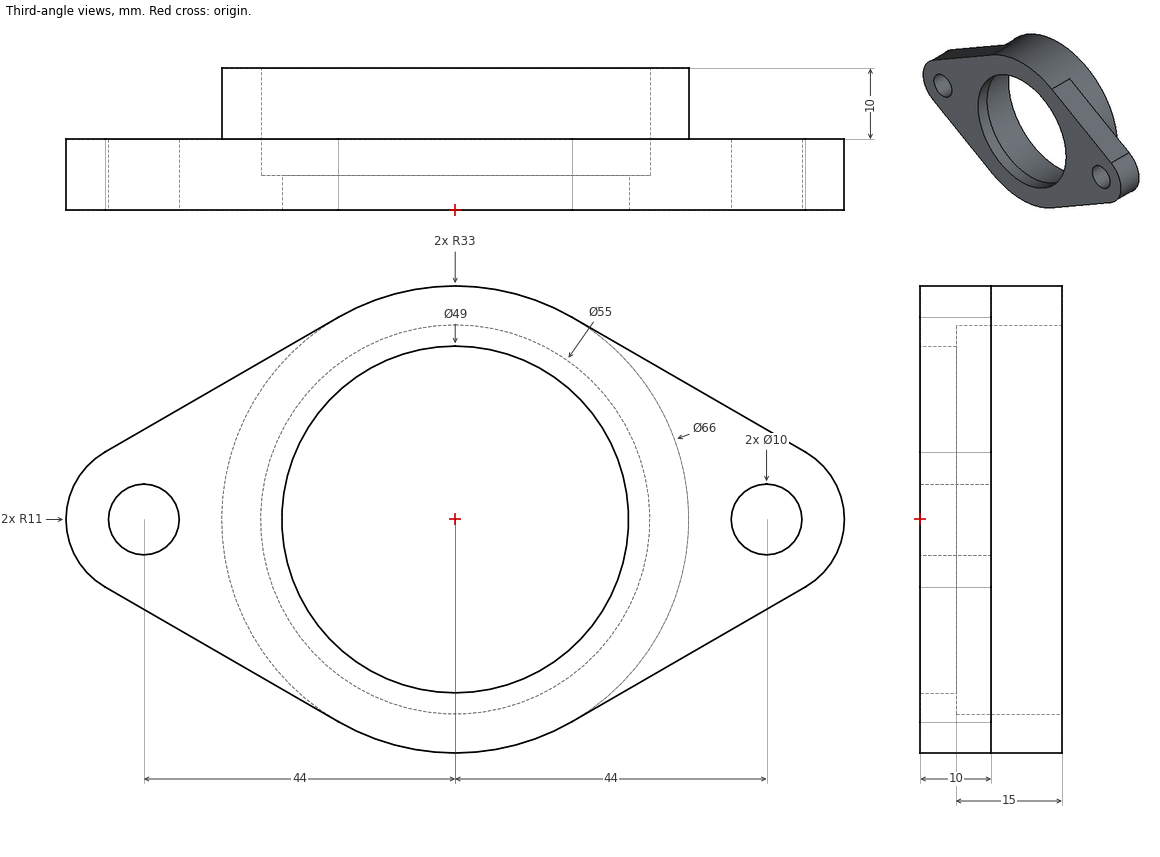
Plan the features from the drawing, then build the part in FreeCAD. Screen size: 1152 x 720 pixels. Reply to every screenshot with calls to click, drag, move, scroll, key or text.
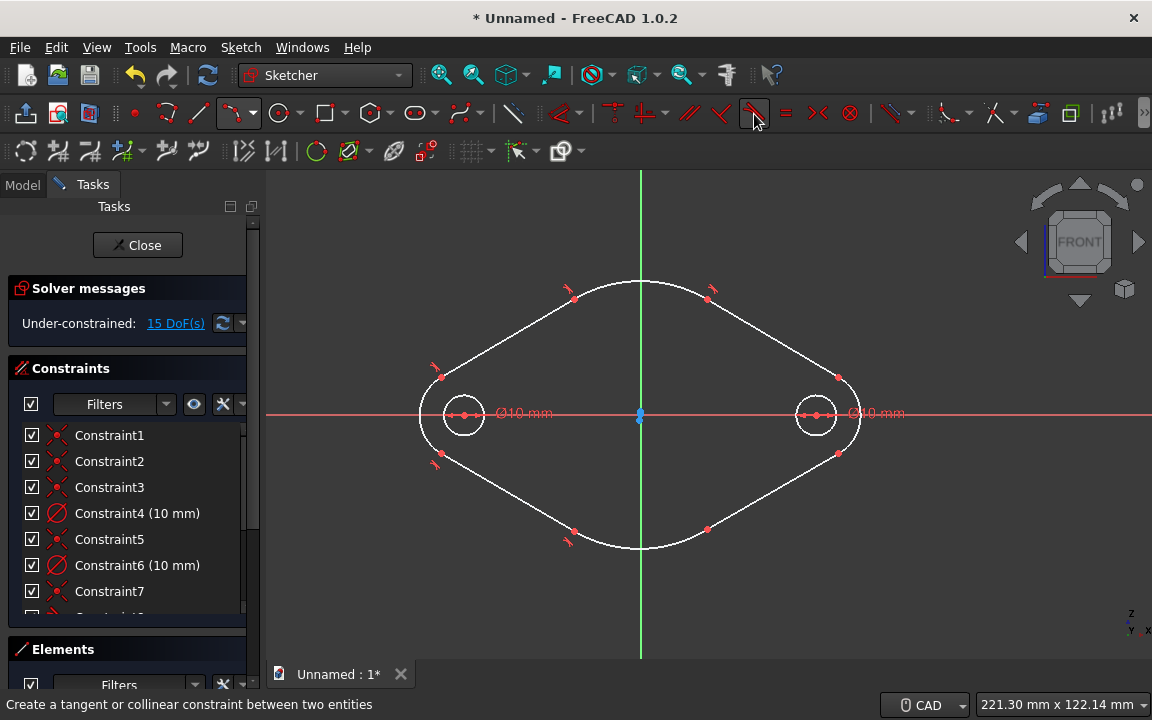
click(746, 323)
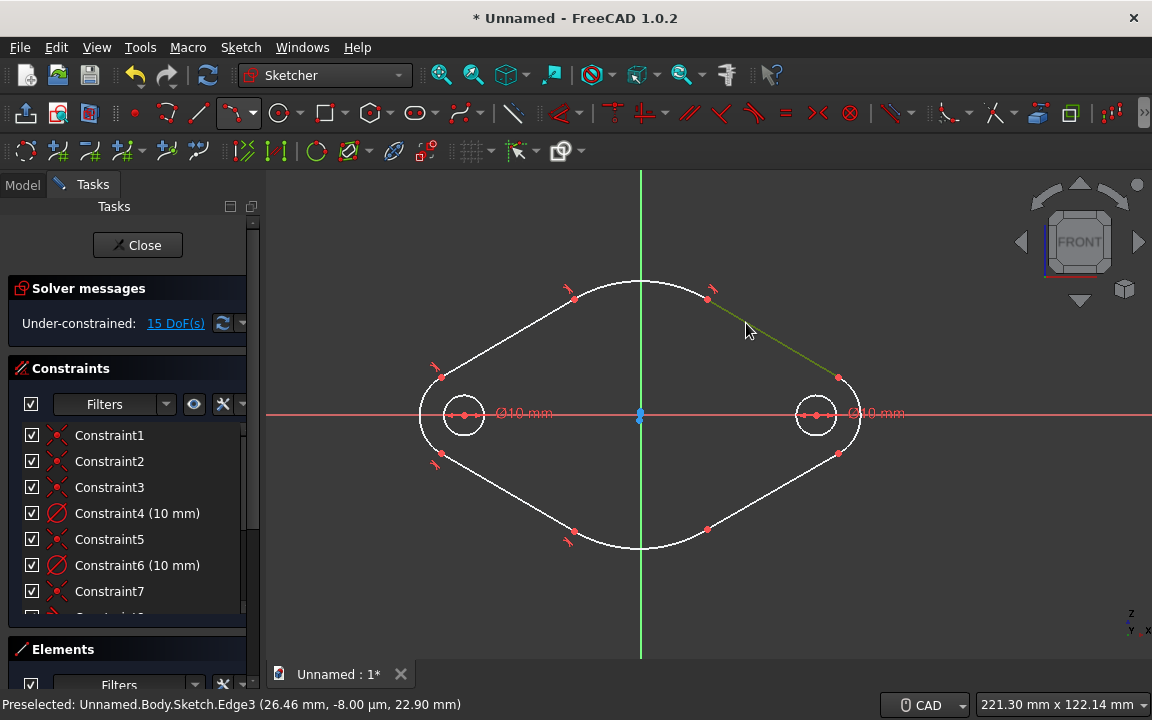
click(857, 434)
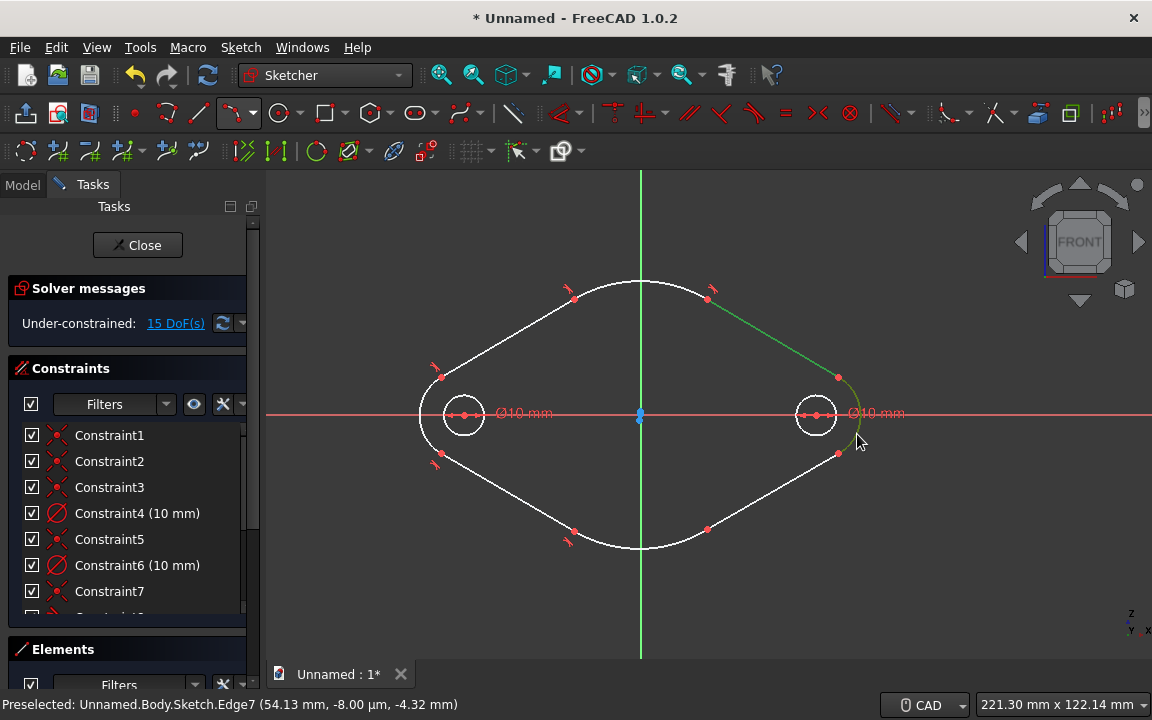
click(754, 114)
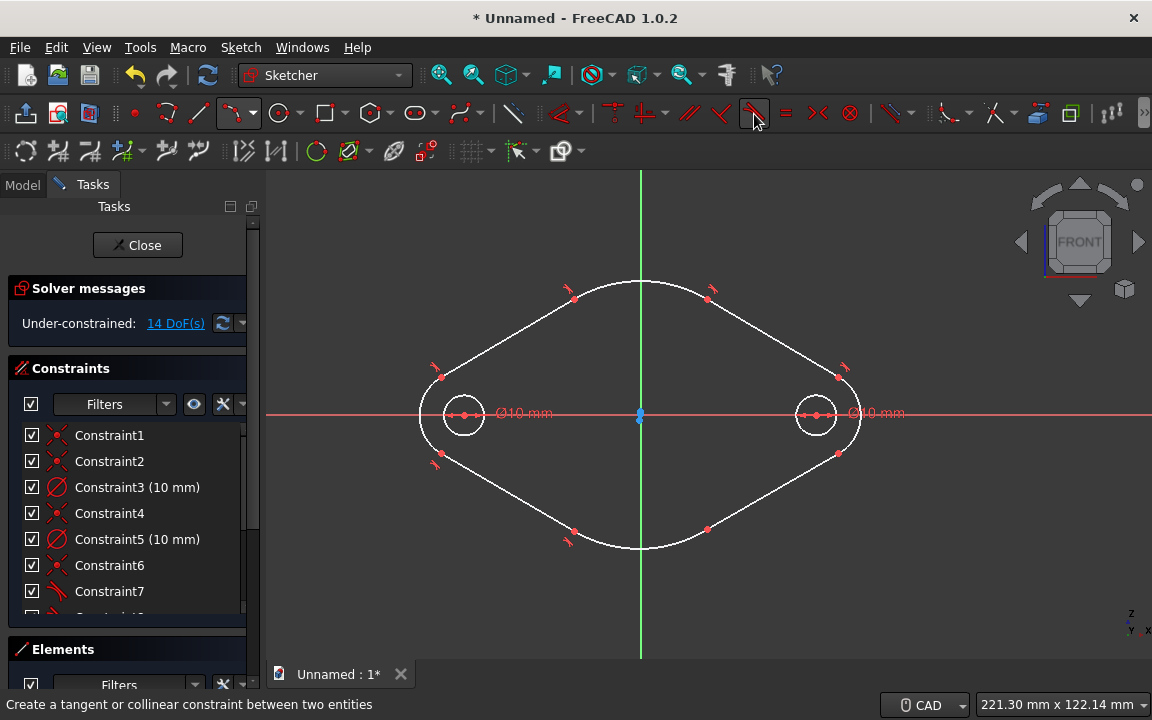
click(799, 477)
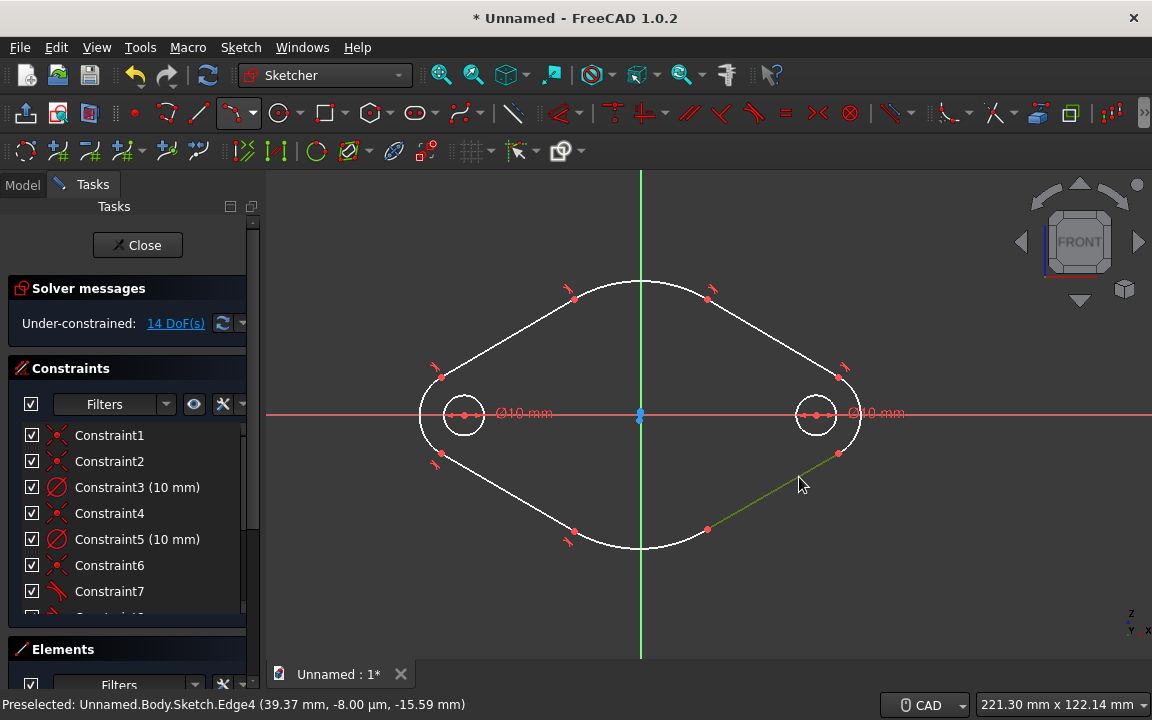
click(857, 434)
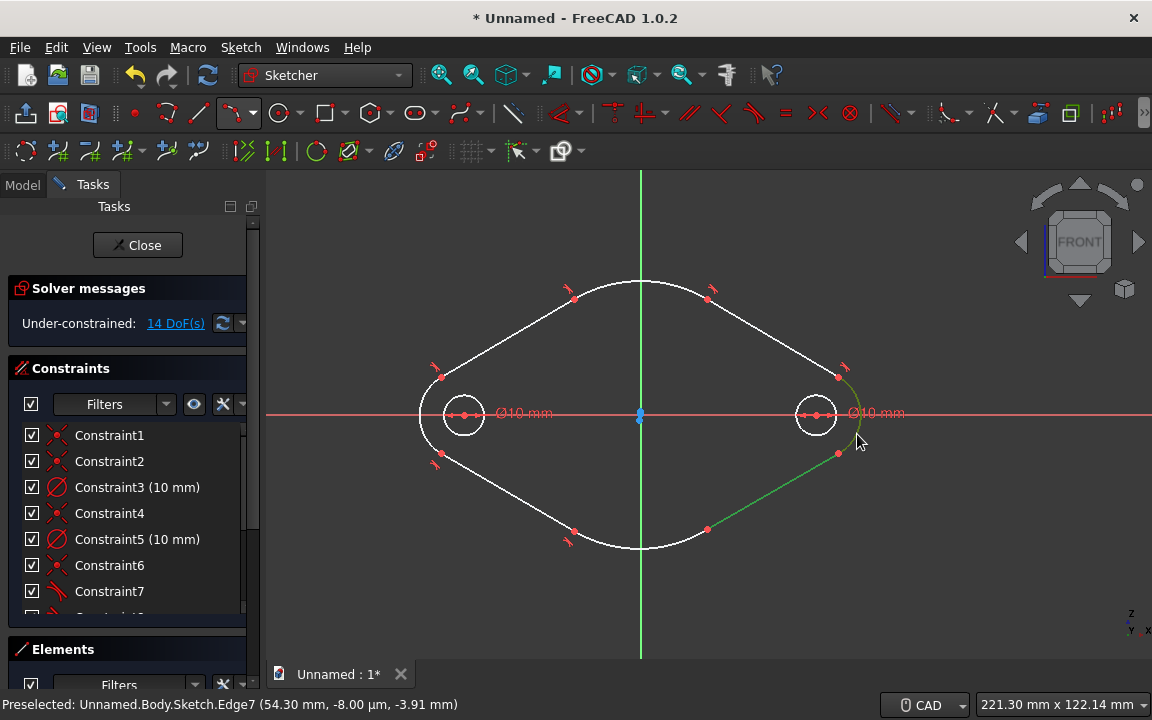
click(754, 114)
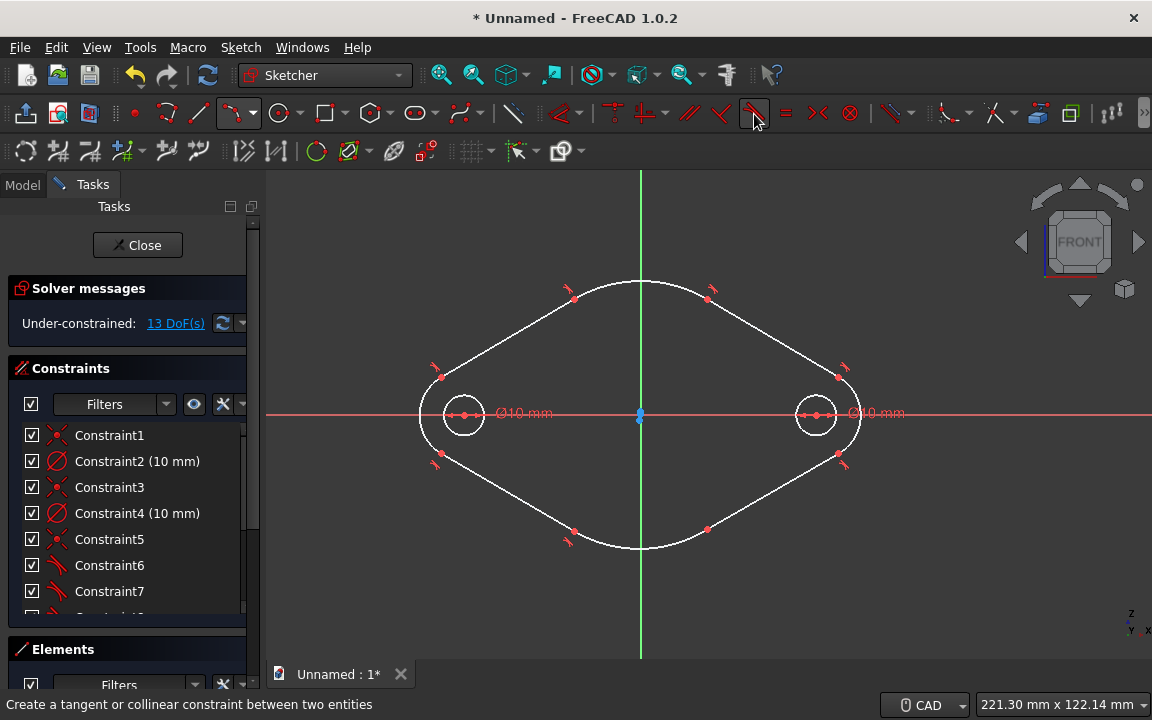
click(799, 477)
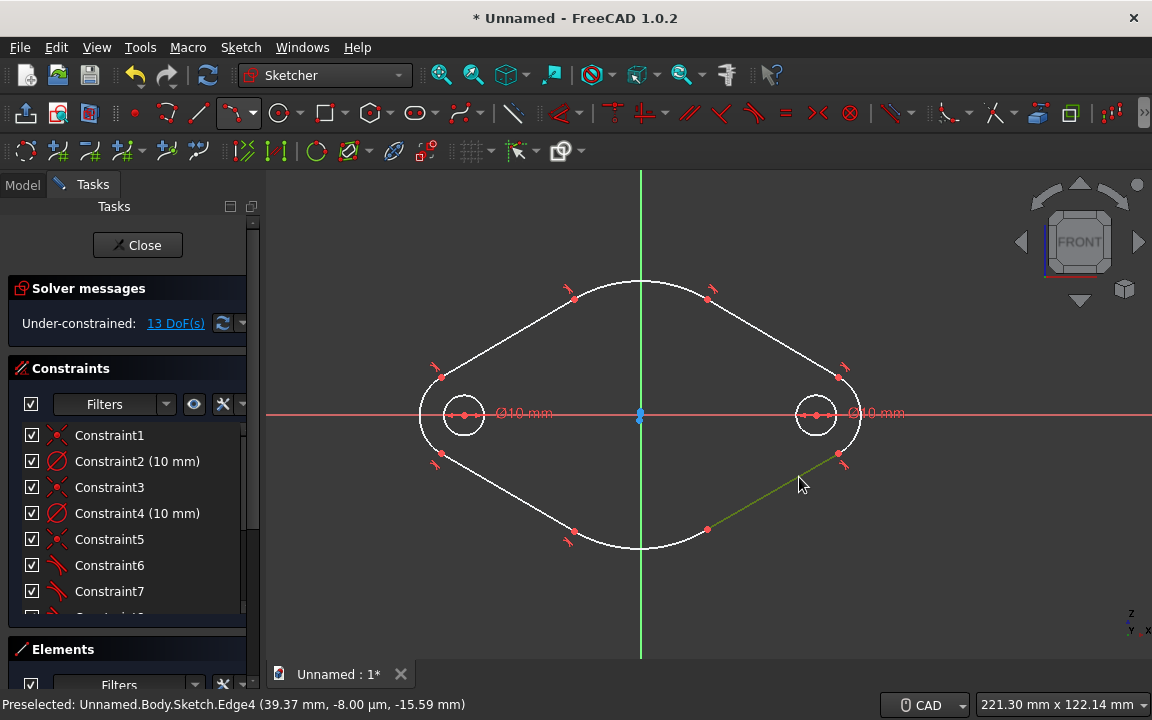
click(613, 546)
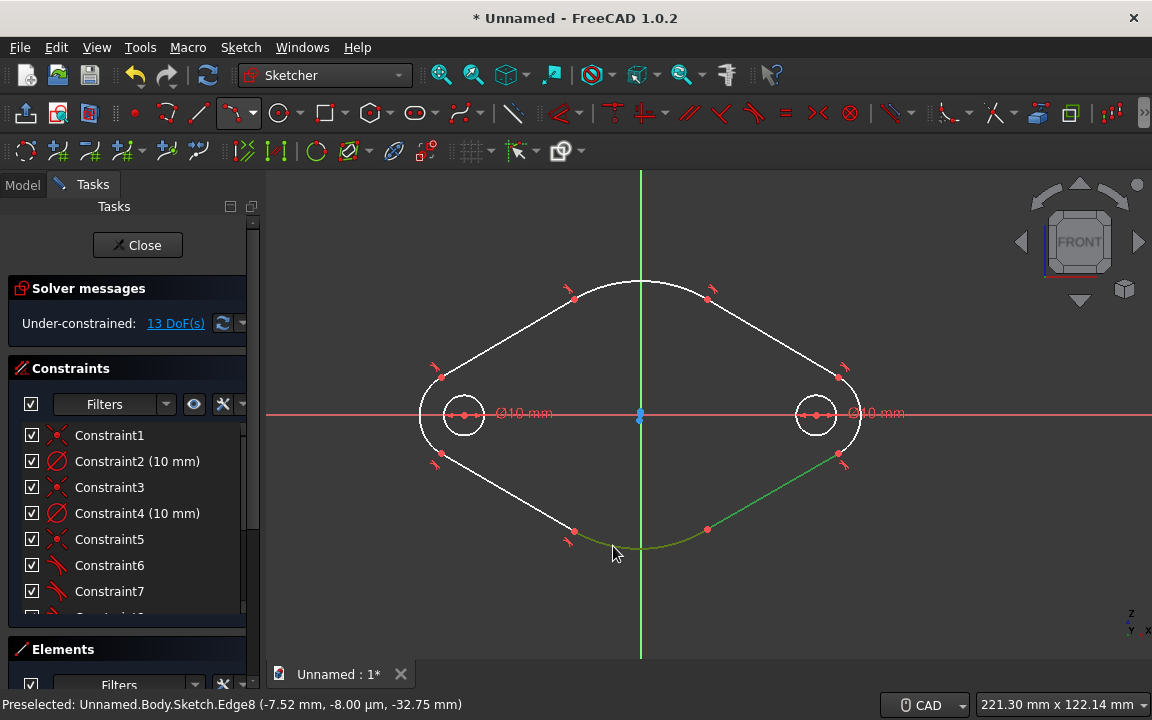
click(754, 114)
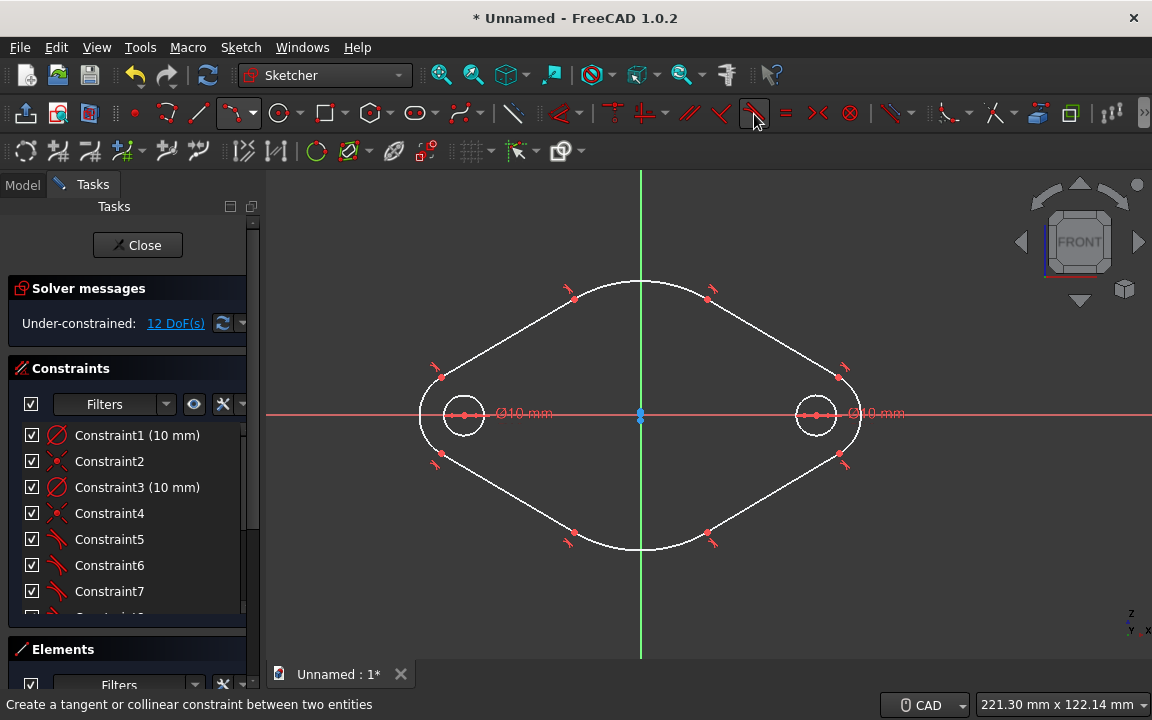
click(668, 284)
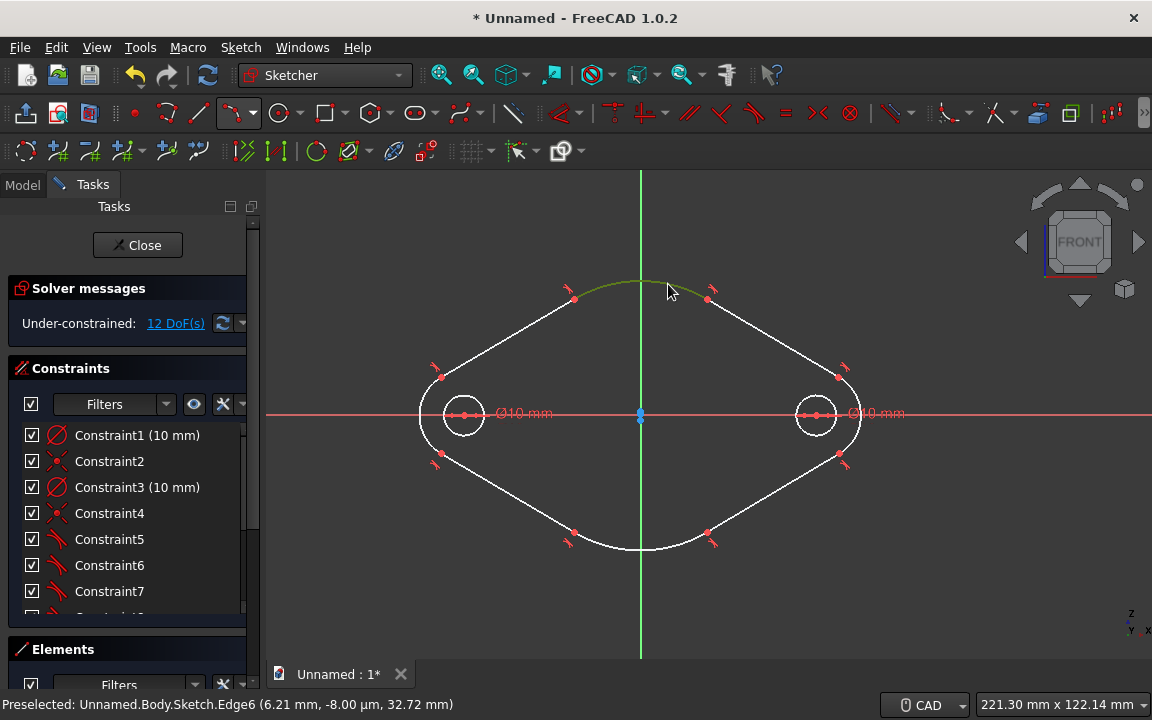
click(613, 548)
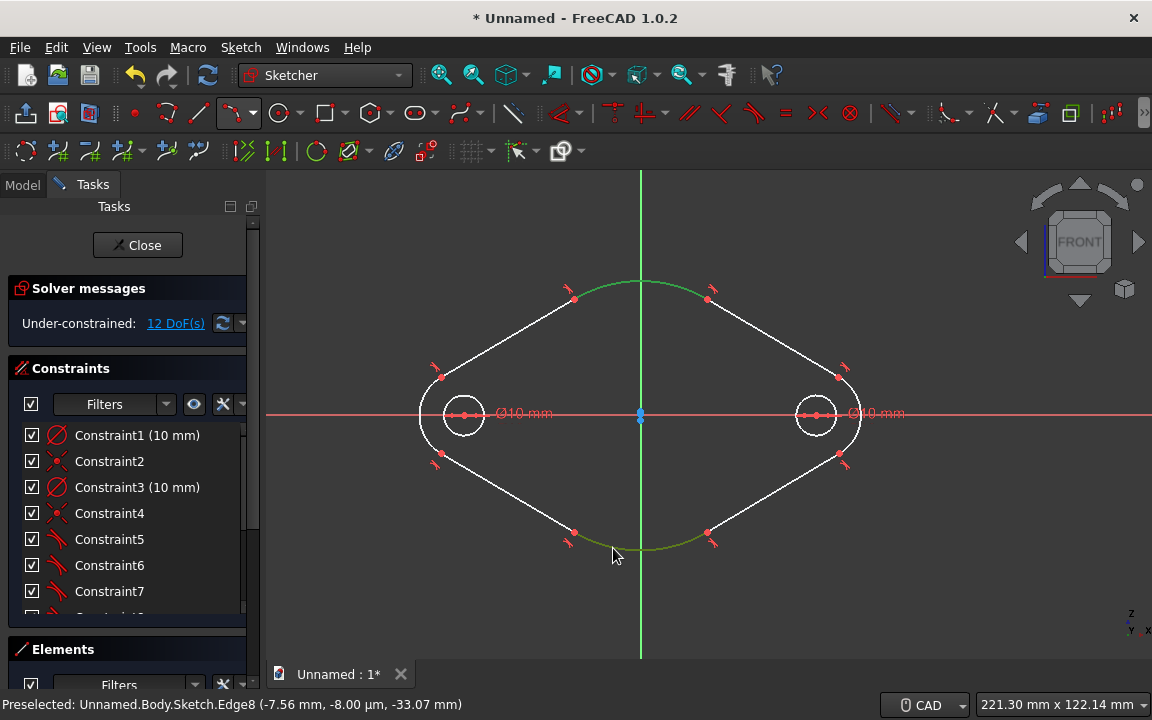
click(614, 114)